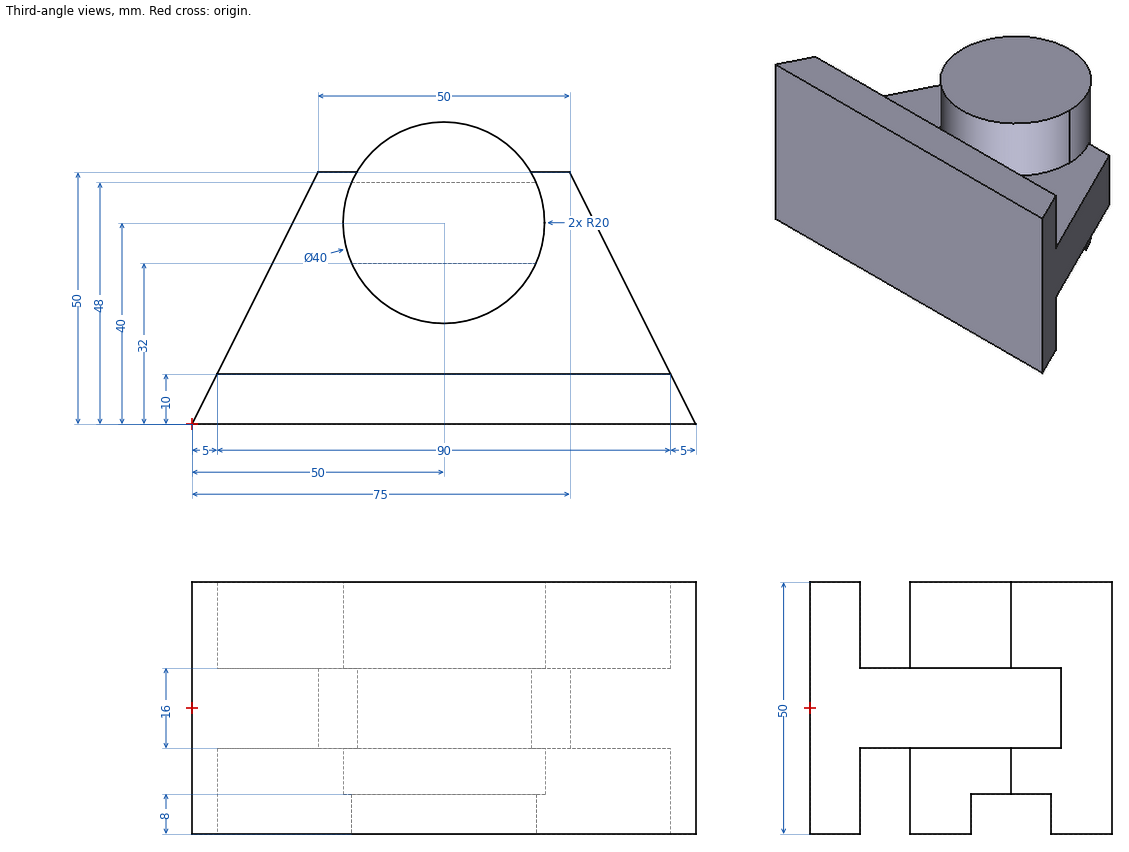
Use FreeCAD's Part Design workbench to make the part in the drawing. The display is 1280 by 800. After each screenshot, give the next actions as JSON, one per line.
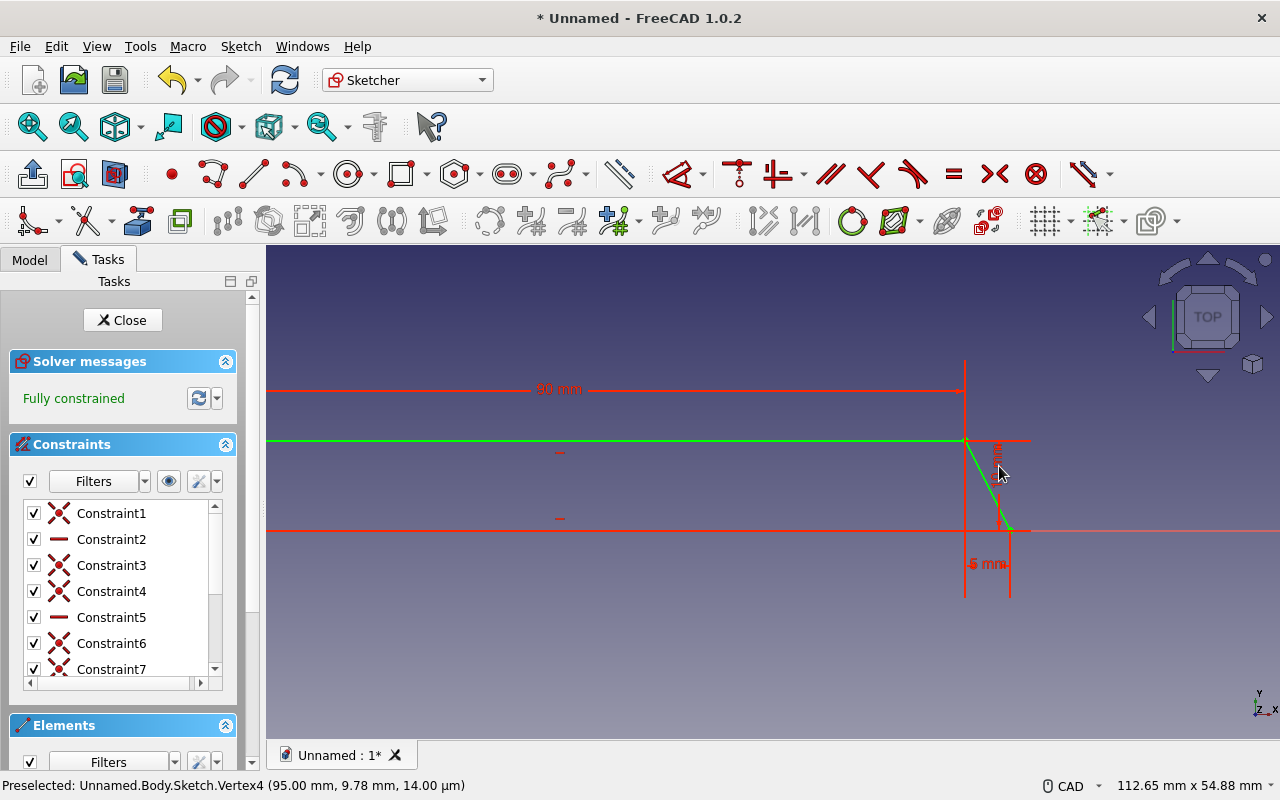
{"action": "left_click", "coordinate": [123, 320]}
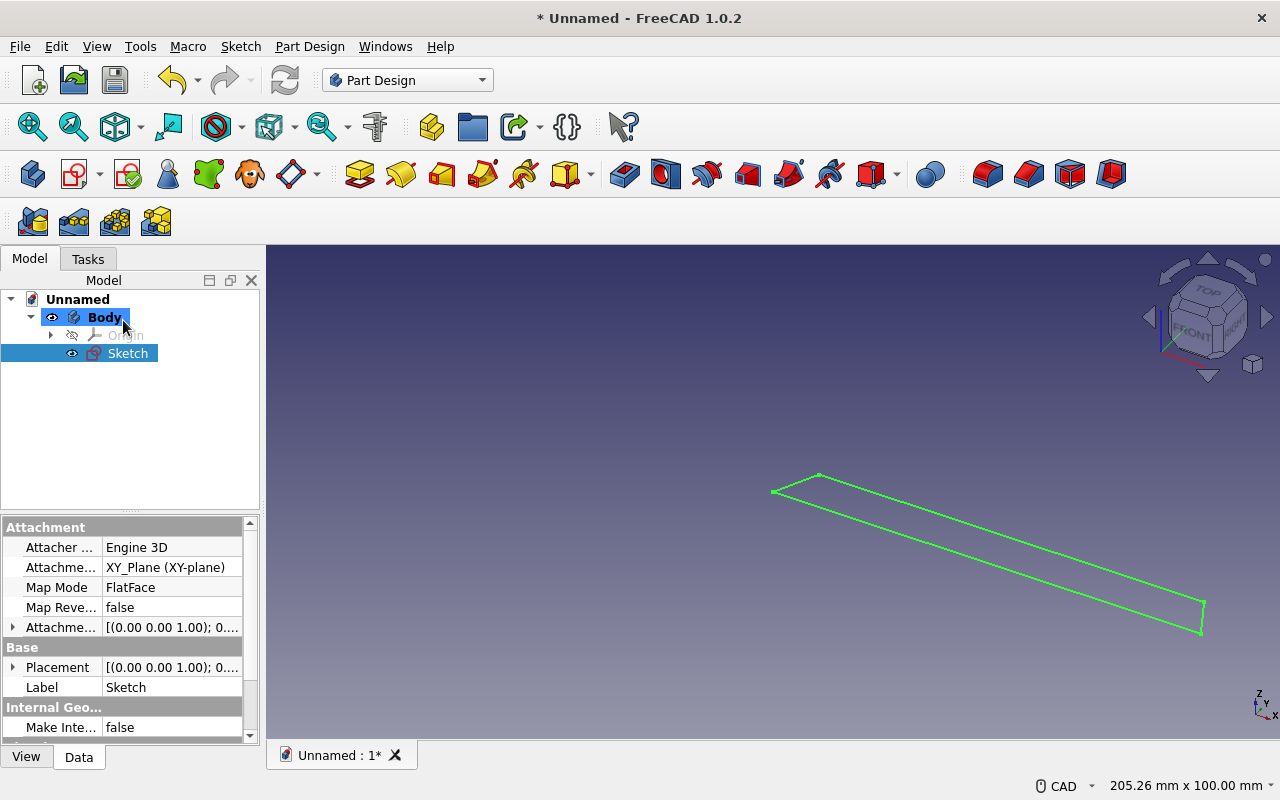
{"action": "left_click", "coordinate": [360, 174]}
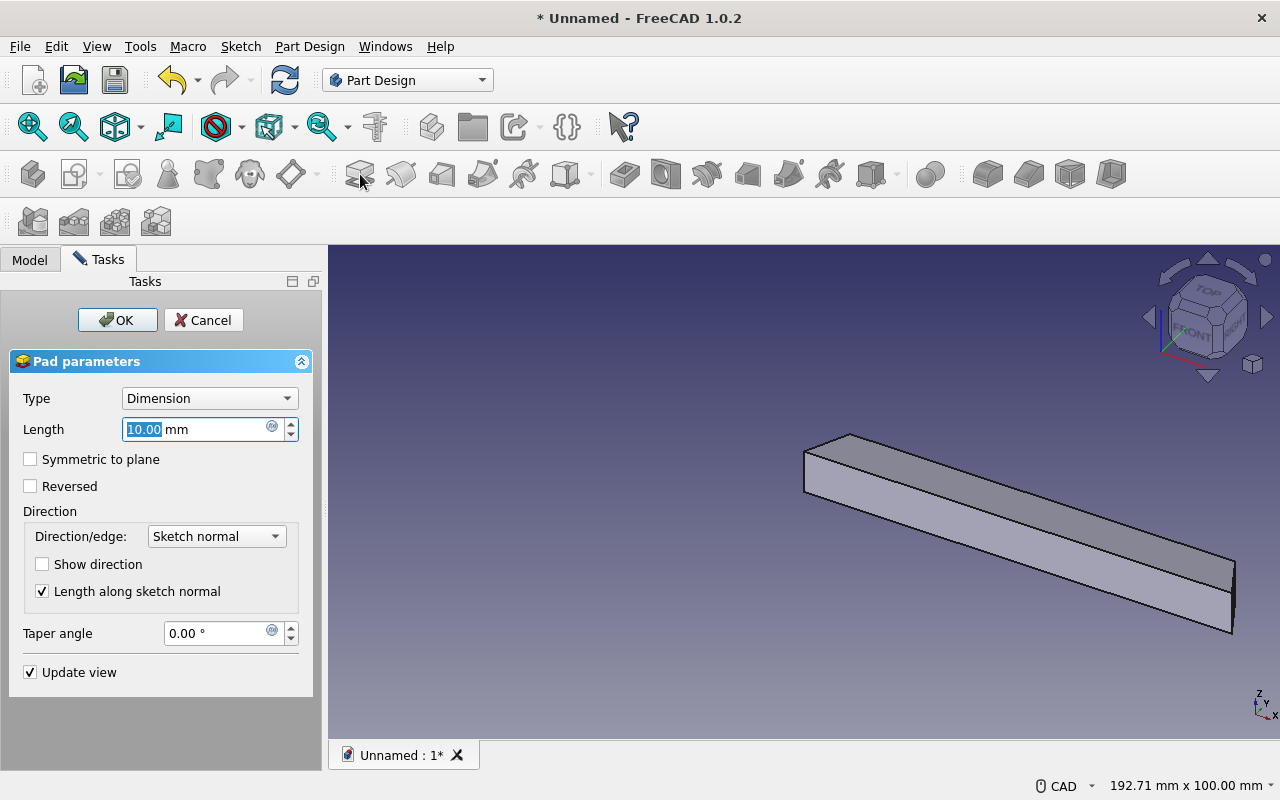
{"action": "type", "text": "50"}
{"action": "key", "text": "Tab"}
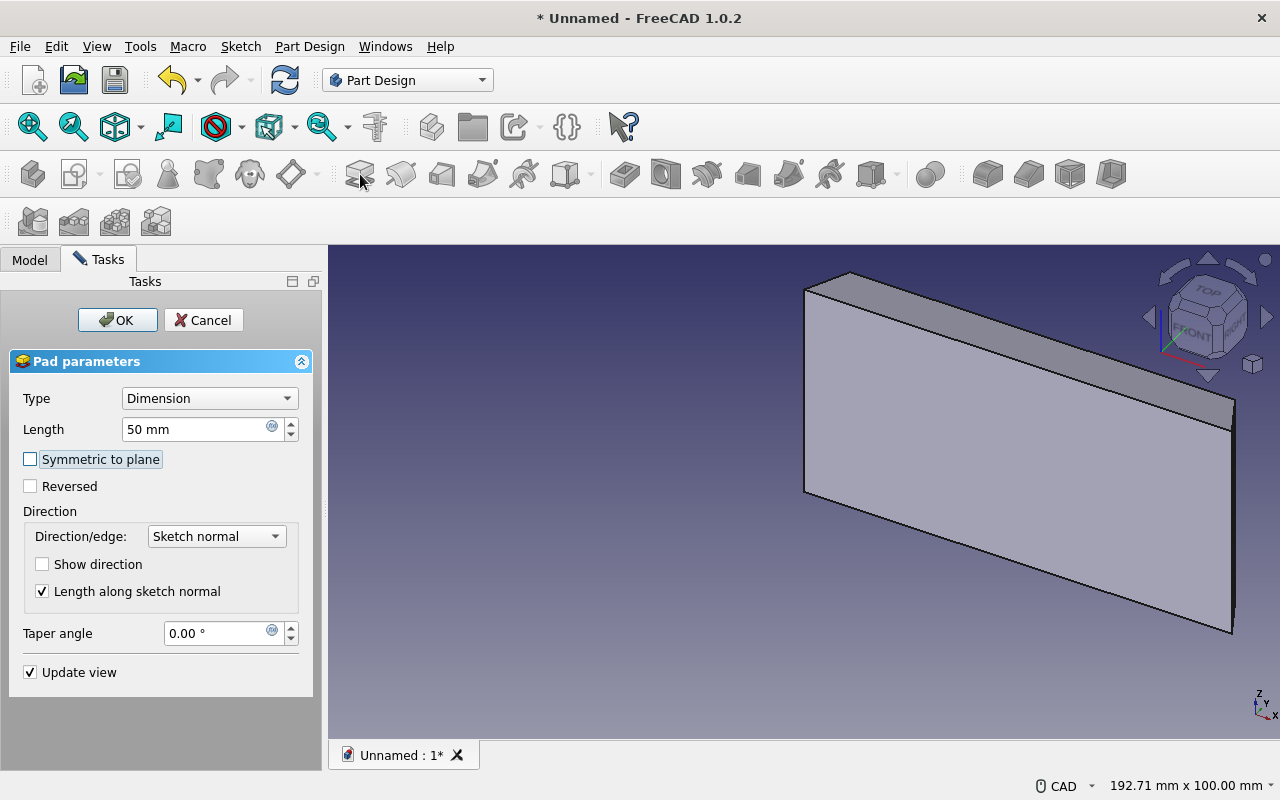
{"action": "left_click", "coordinate": [31, 459]}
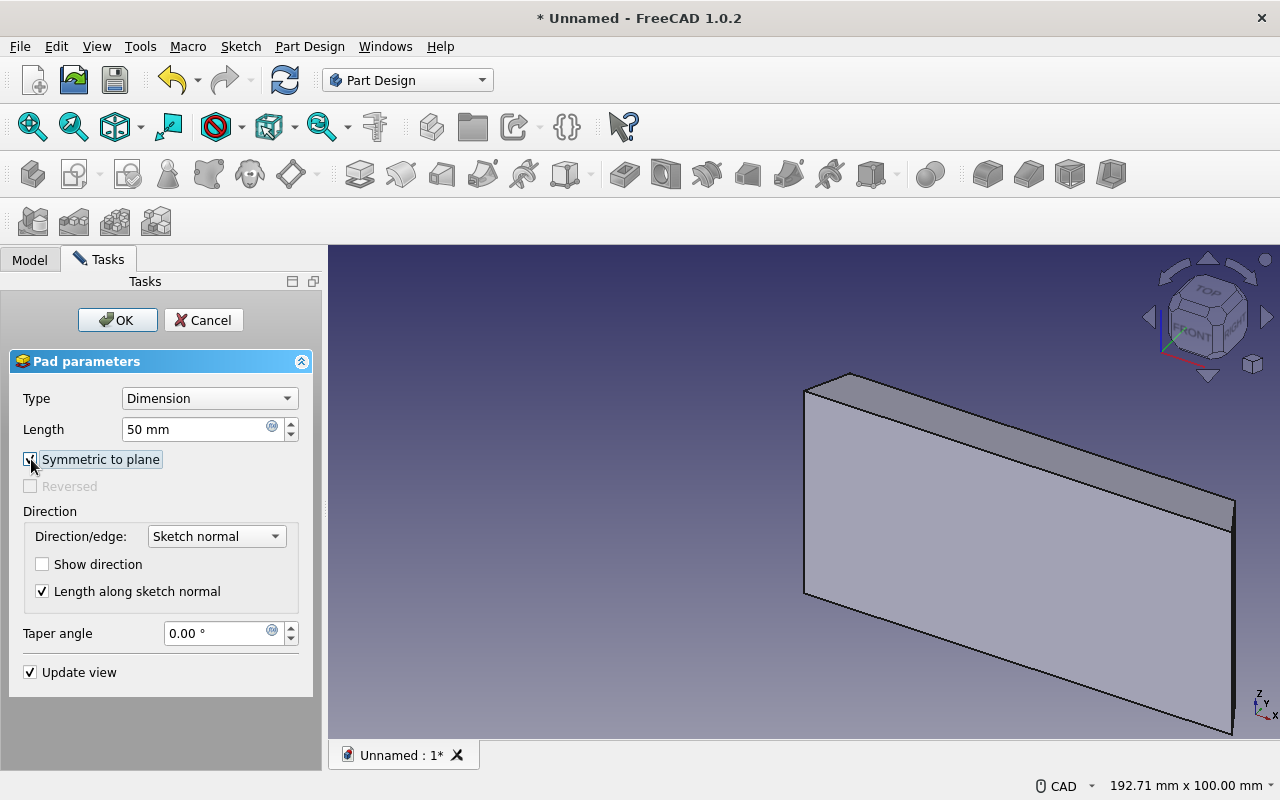
{"action": "left_click", "coordinate": [118, 320]}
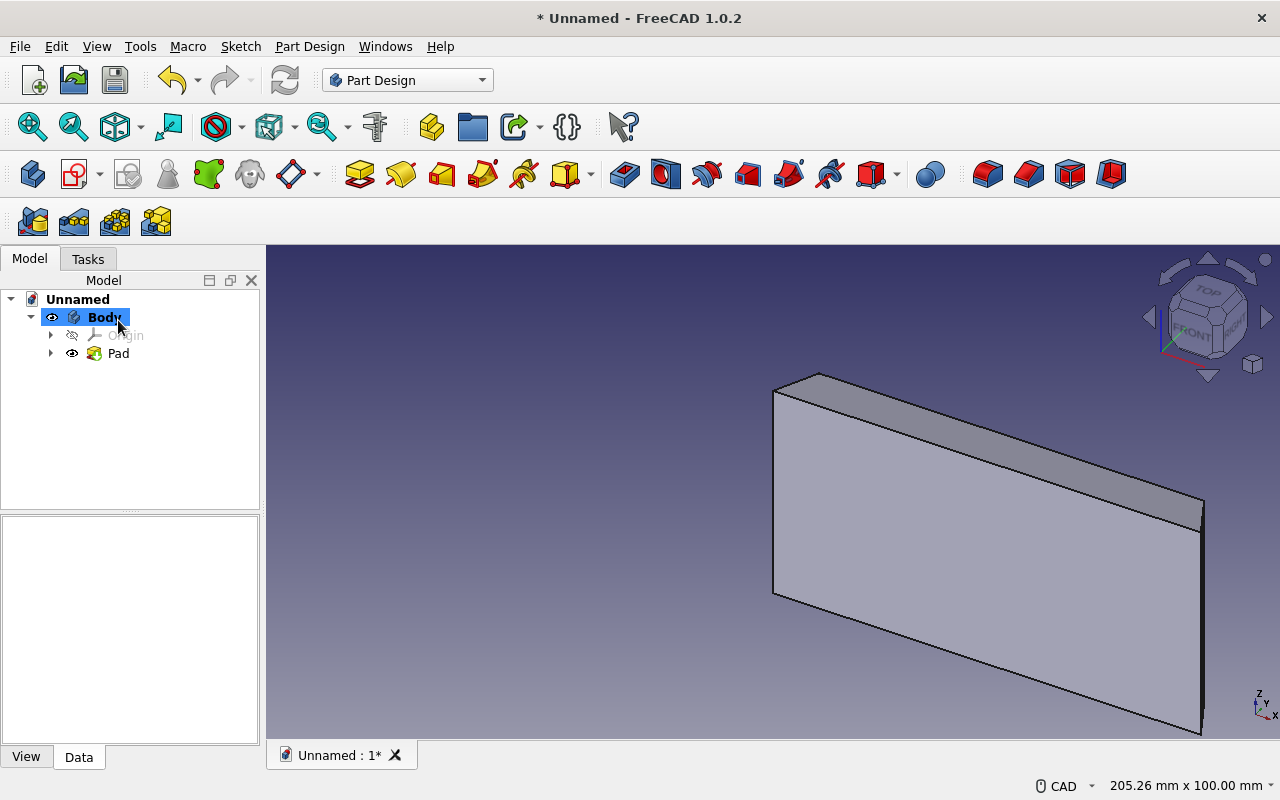
{"action": "left_click", "coordinate": [74, 174]}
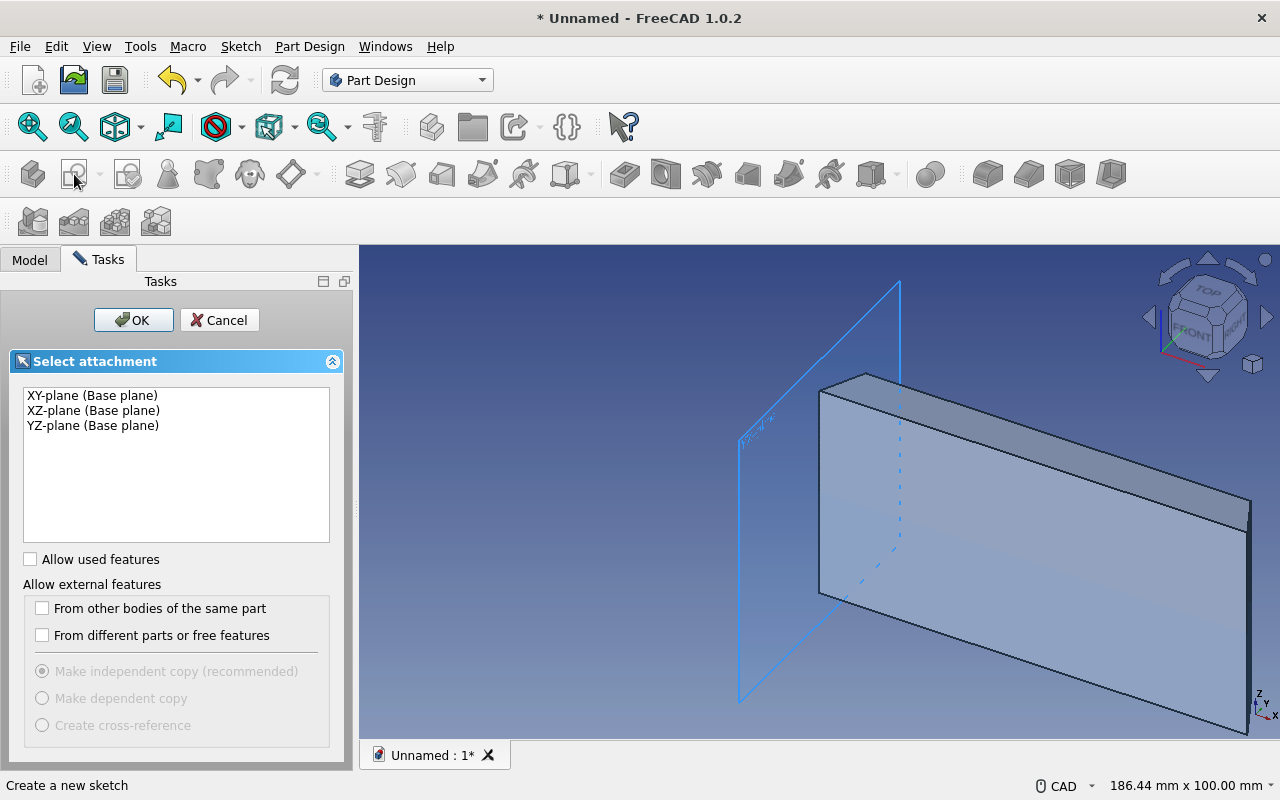
{"action": "left_click", "coordinate": [84, 396]}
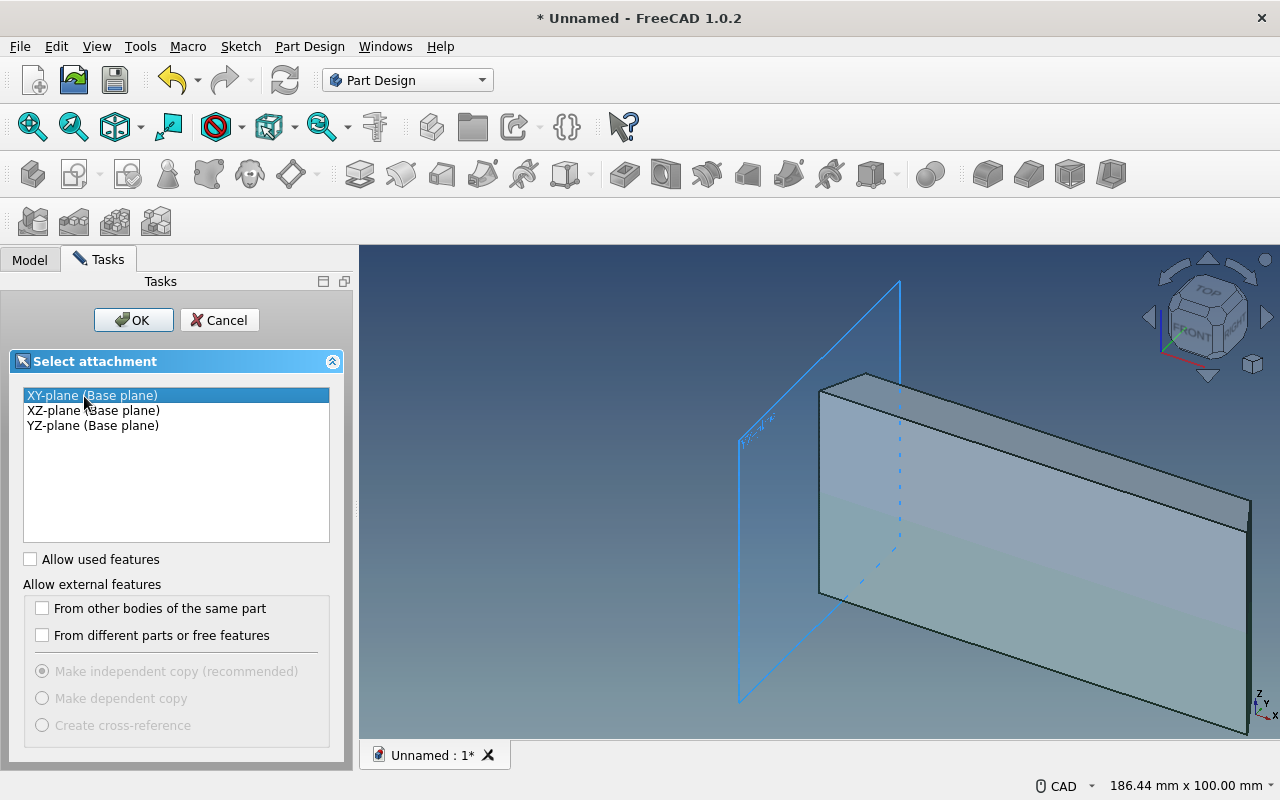
{"action": "left_click", "coordinate": [134, 320]}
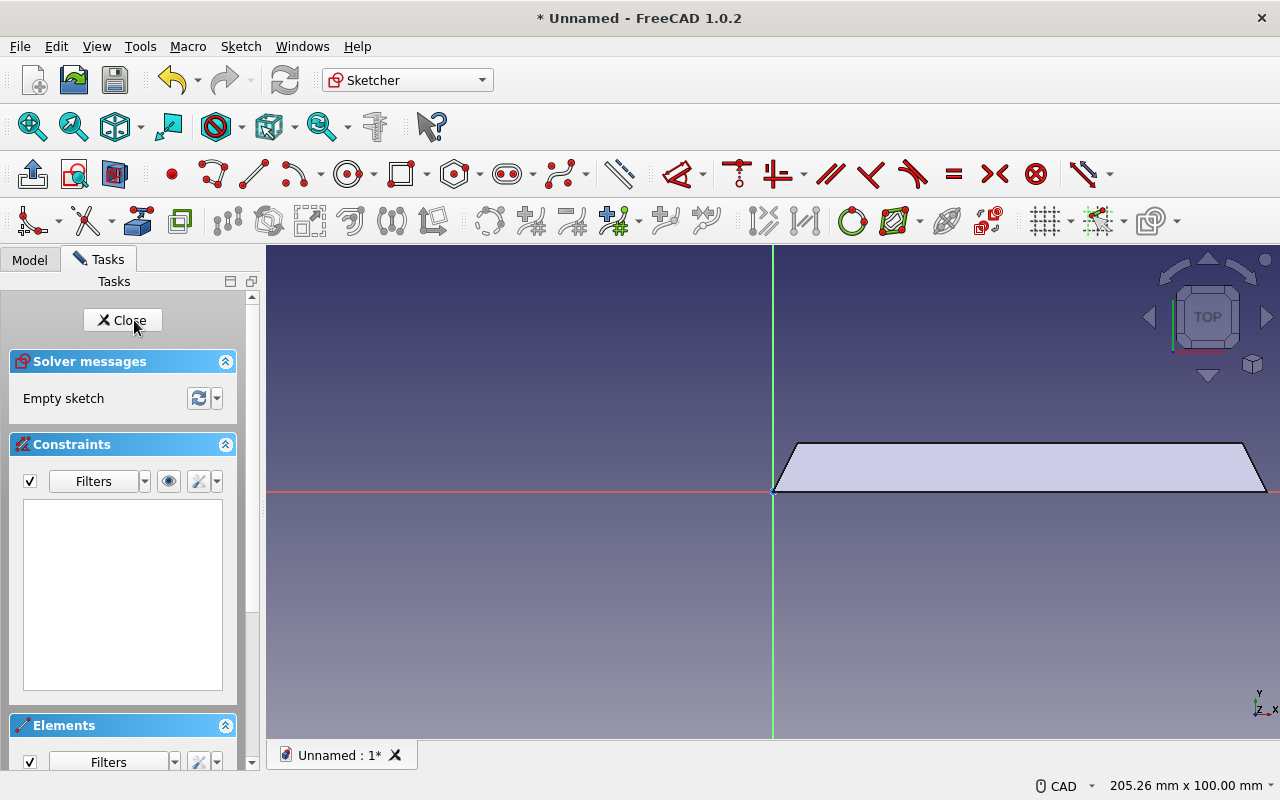
{"action": "left_click", "coordinate": [115, 174]}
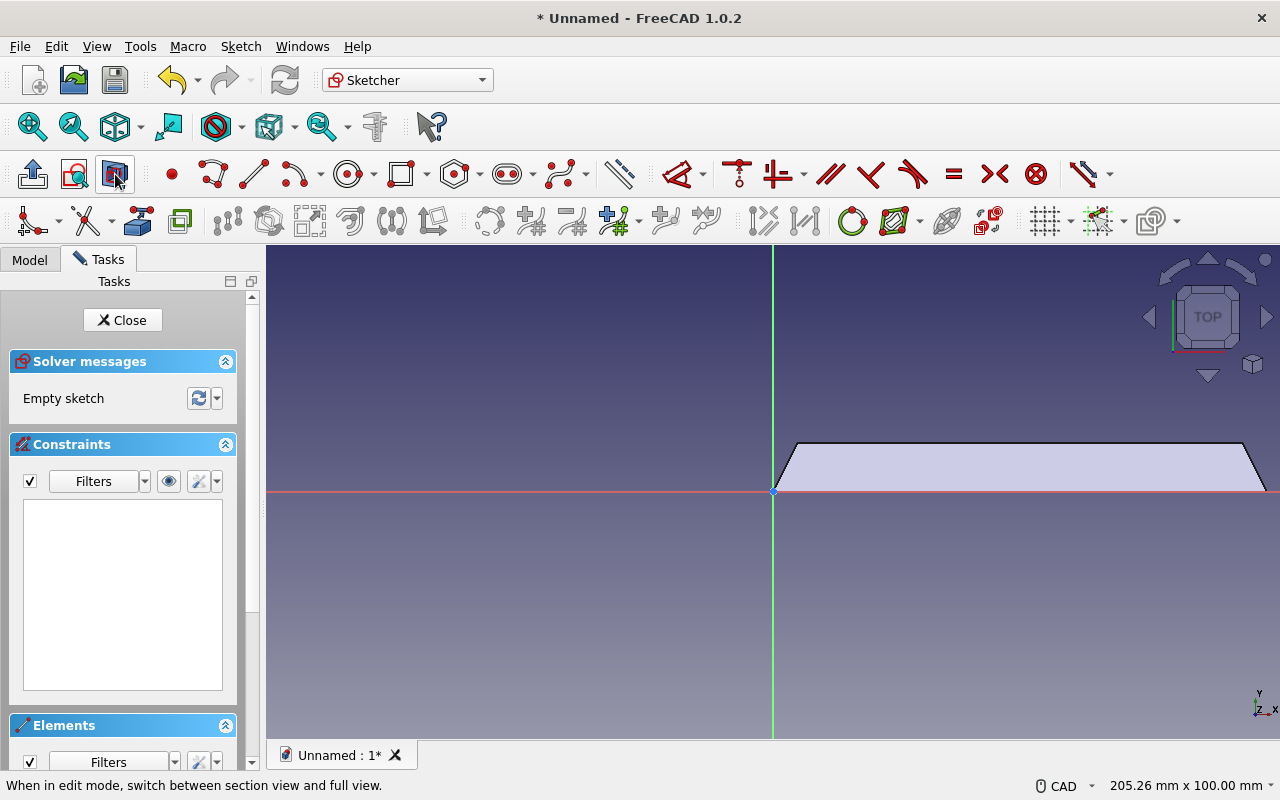
{"action": "scroll", "coordinate": [294, 711], "scroll_direction": "down", "scroll_amount": 1}